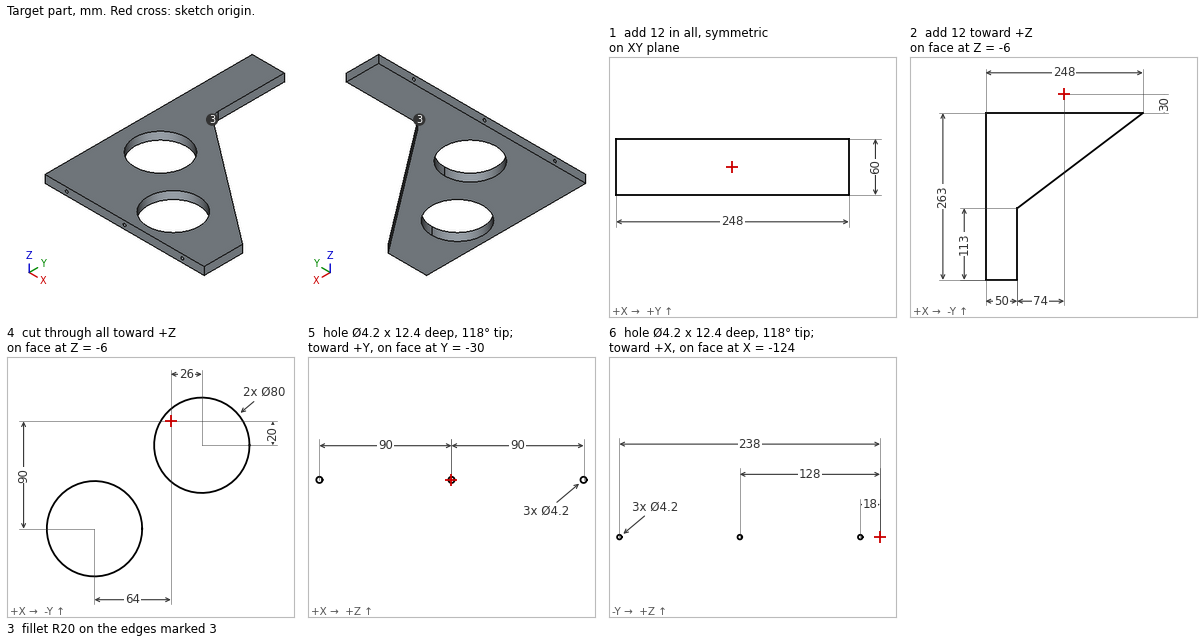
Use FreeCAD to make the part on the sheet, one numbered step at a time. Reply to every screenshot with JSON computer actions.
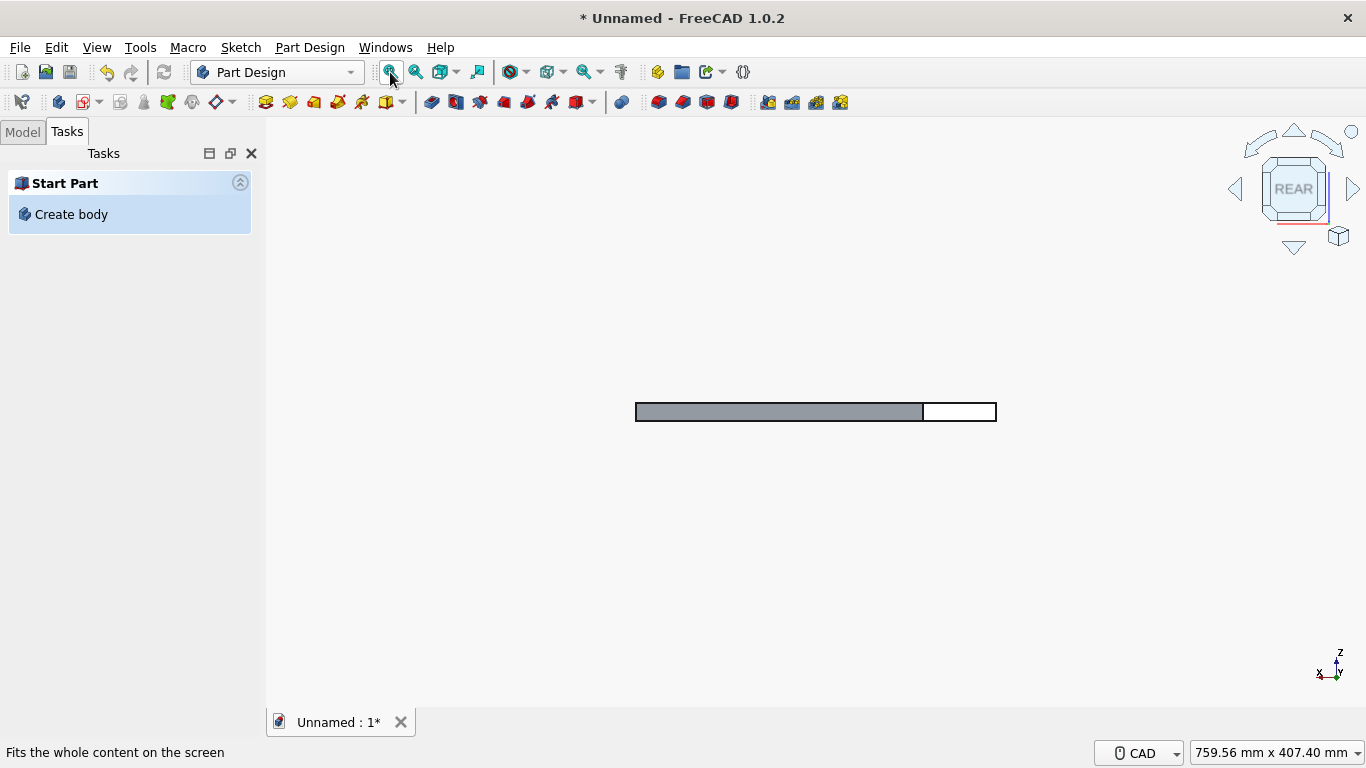
{"action": "scroll", "coordinate": [923, 411], "scroll_direction": "up", "scroll_amount": 5}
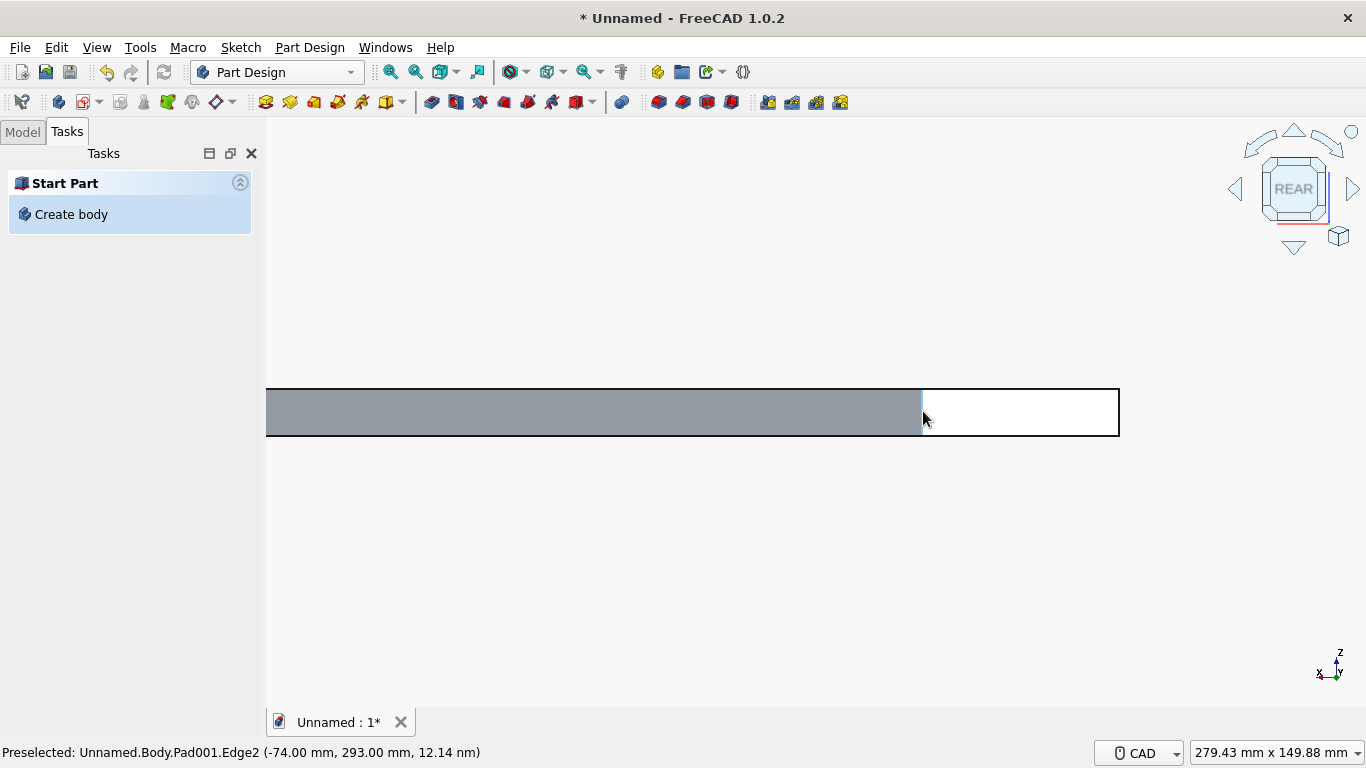
{"action": "left_click", "coordinate": [392, 72]}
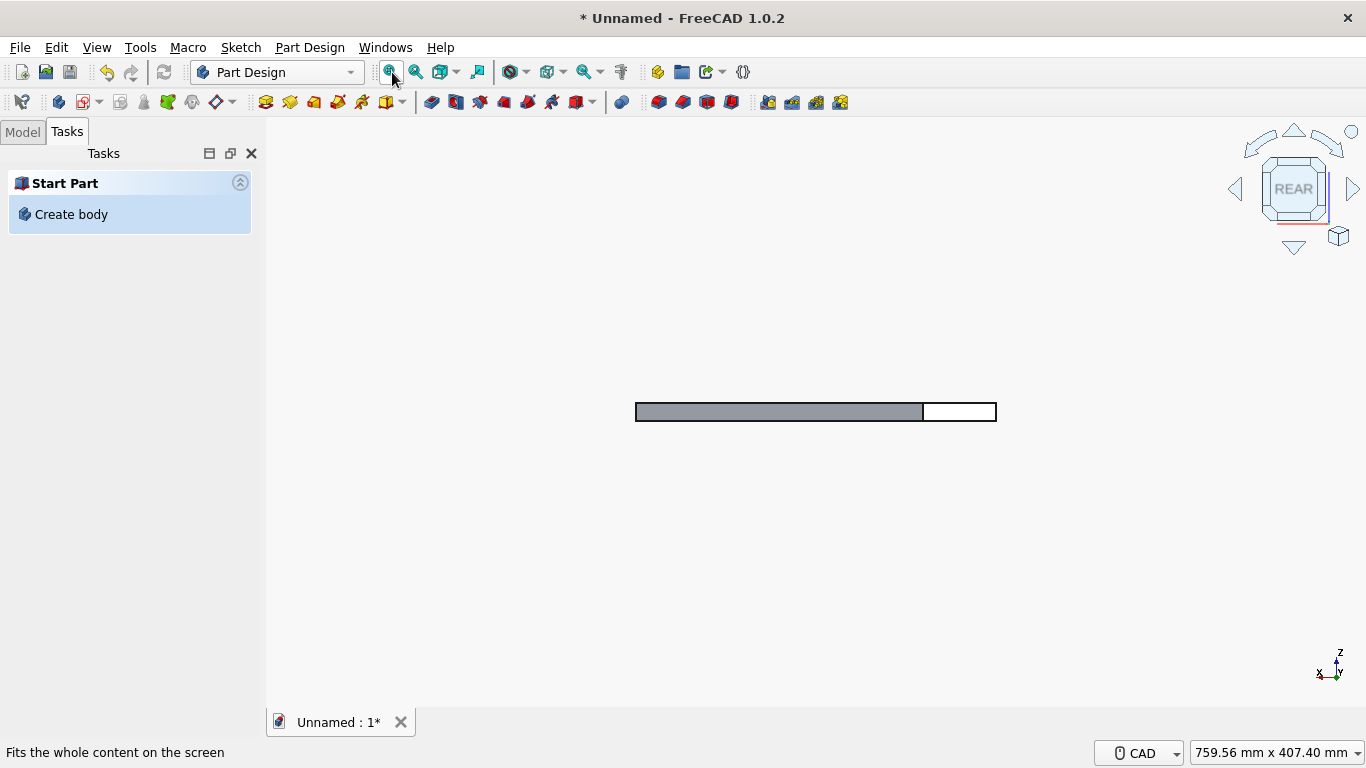
{"action": "key", "text": "6"}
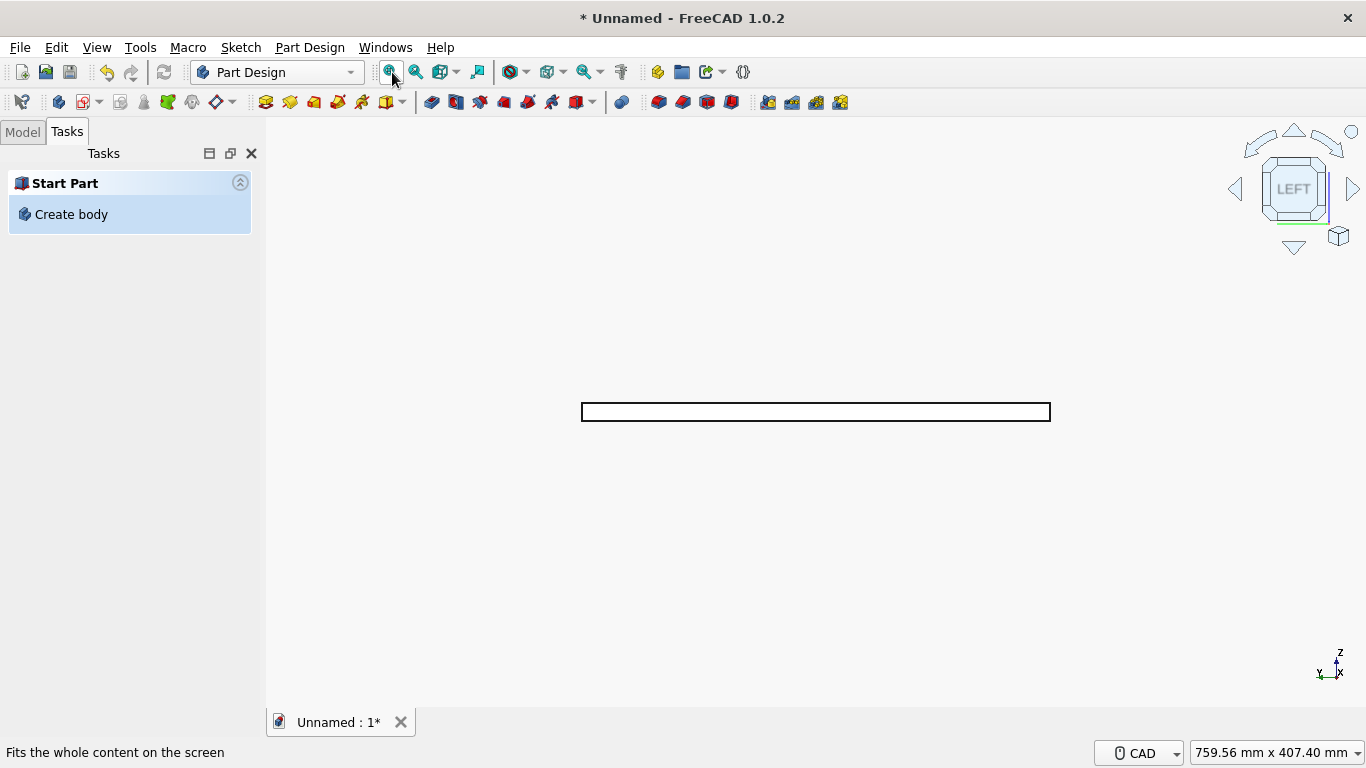
{"action": "key", "text": "v f"}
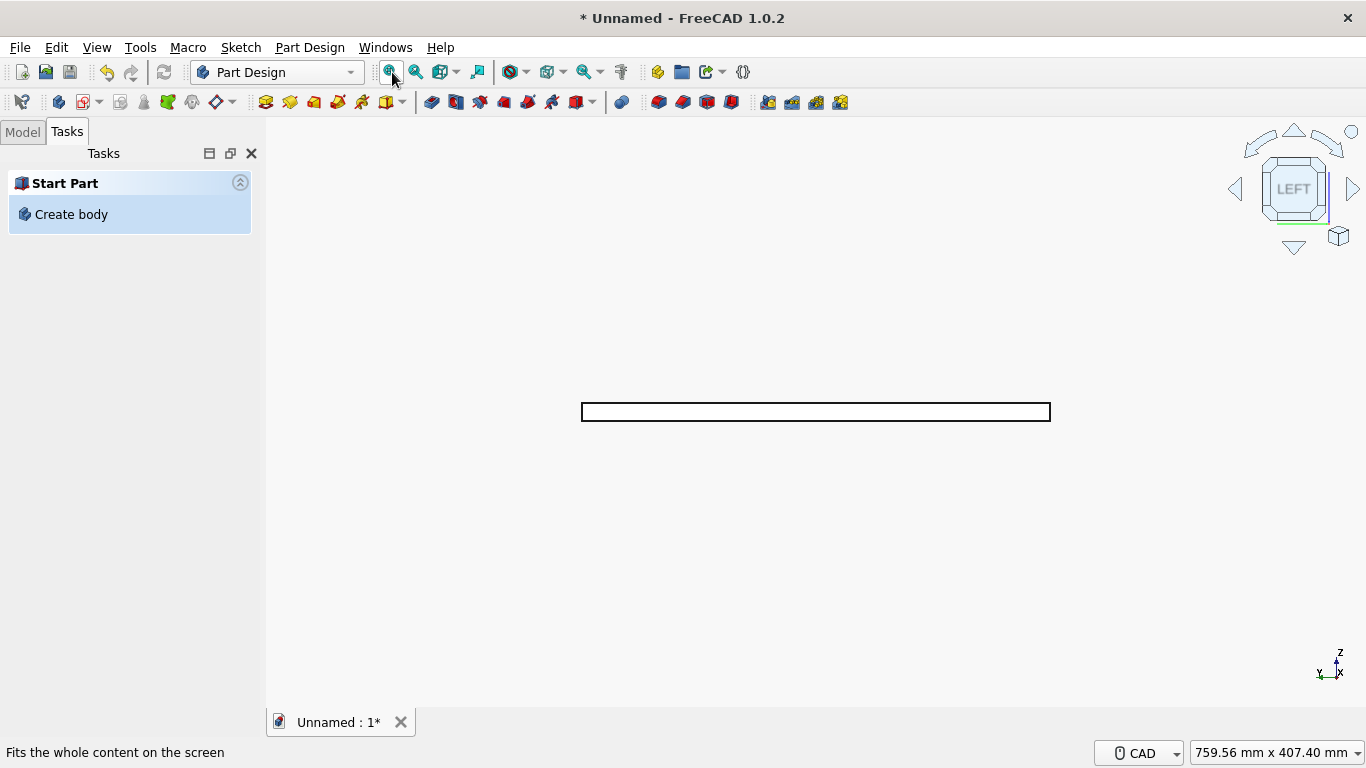
{"action": "scroll", "coordinate": [746, 411], "scroll_direction": "up", "scroll_amount": 5}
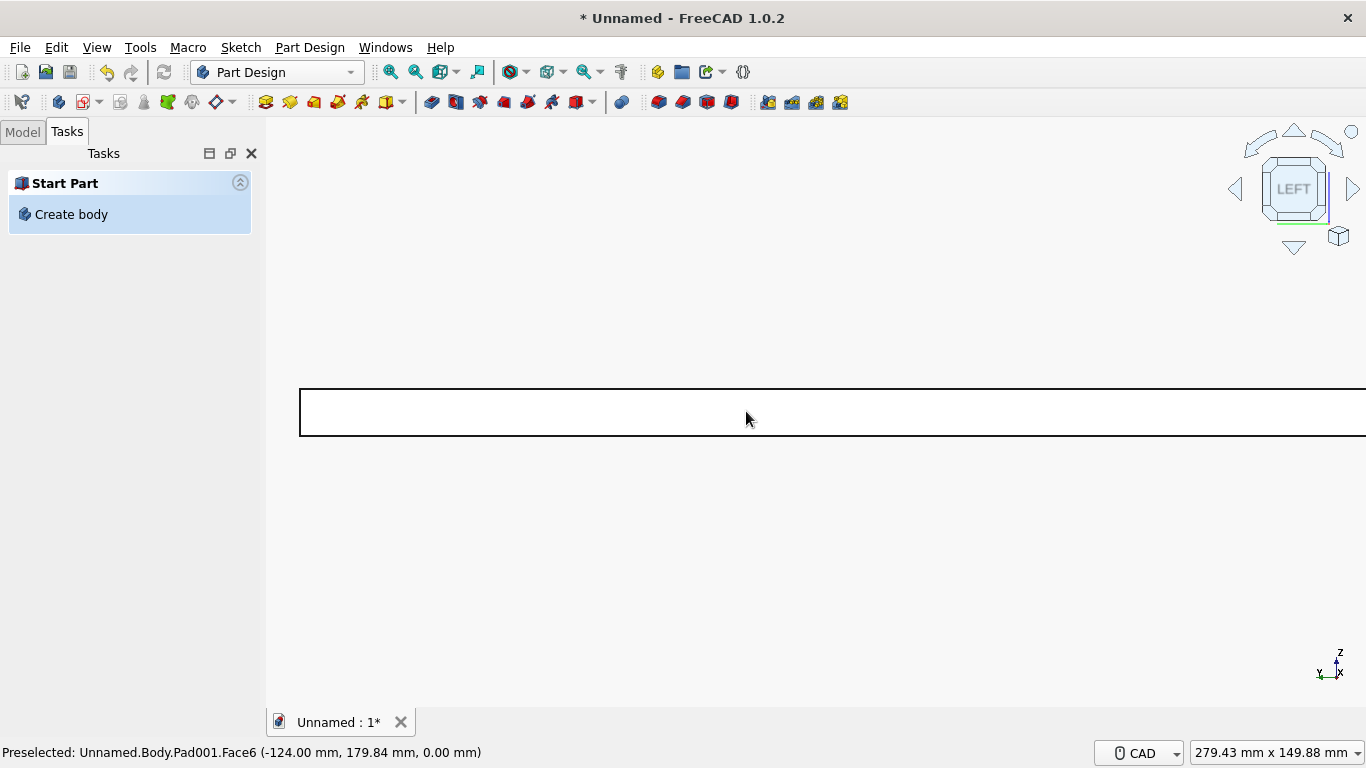
{"action": "key", "text": "v f"}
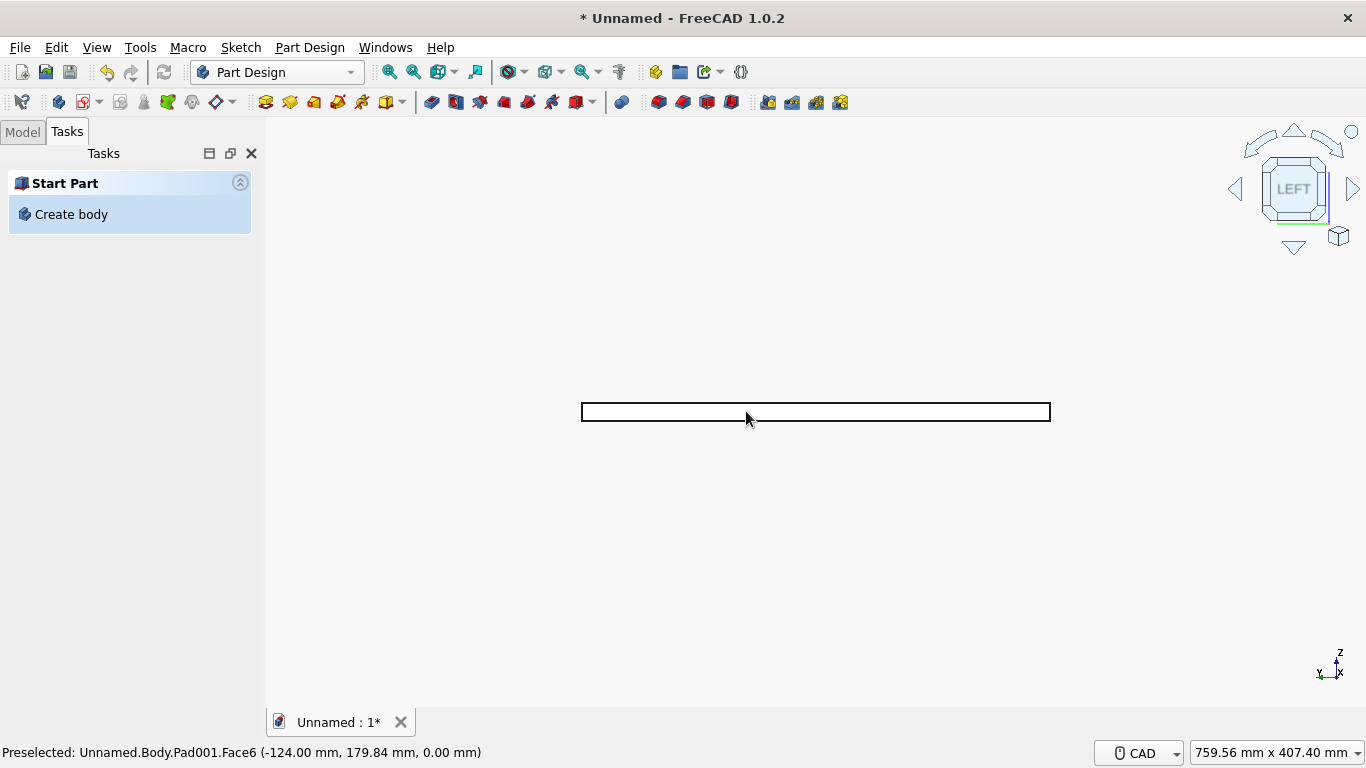
{"action": "key", "text": "v 3"}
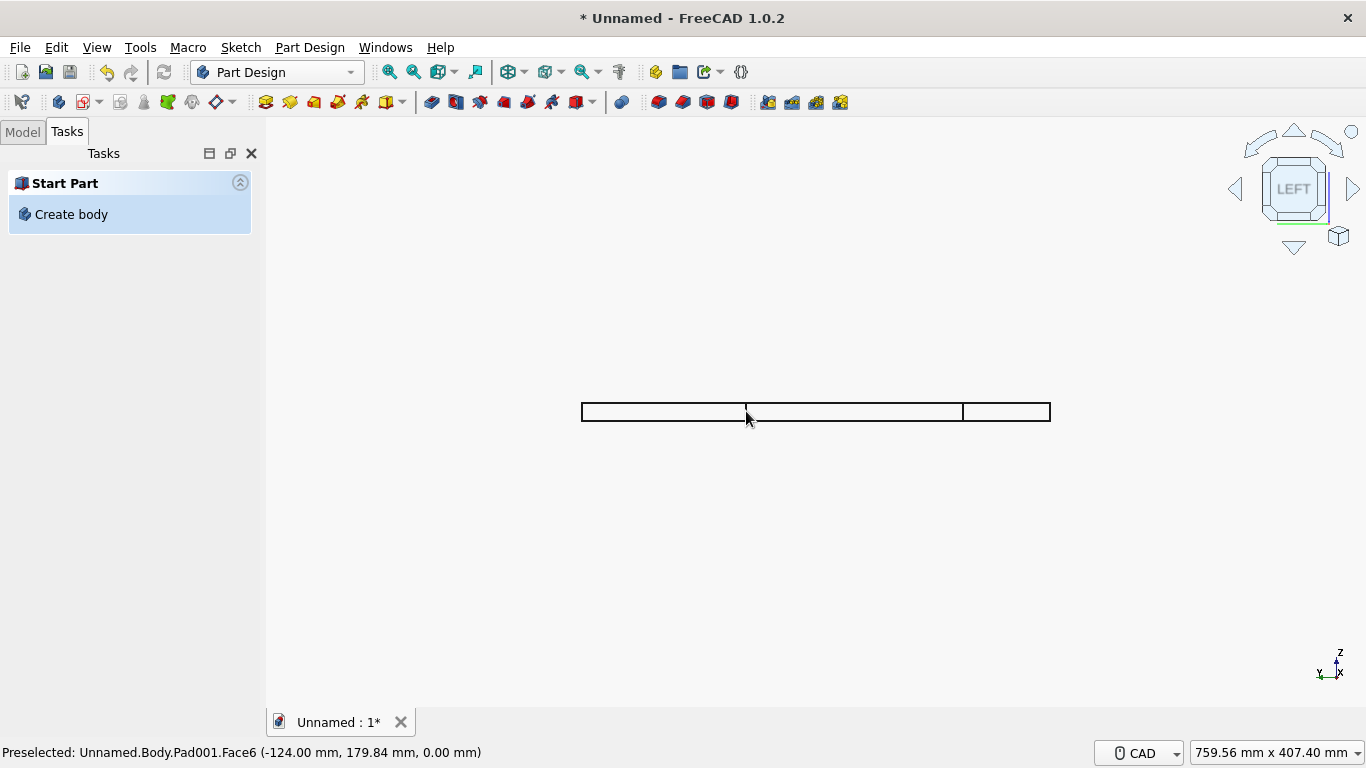
{"action": "key", "text": "0"}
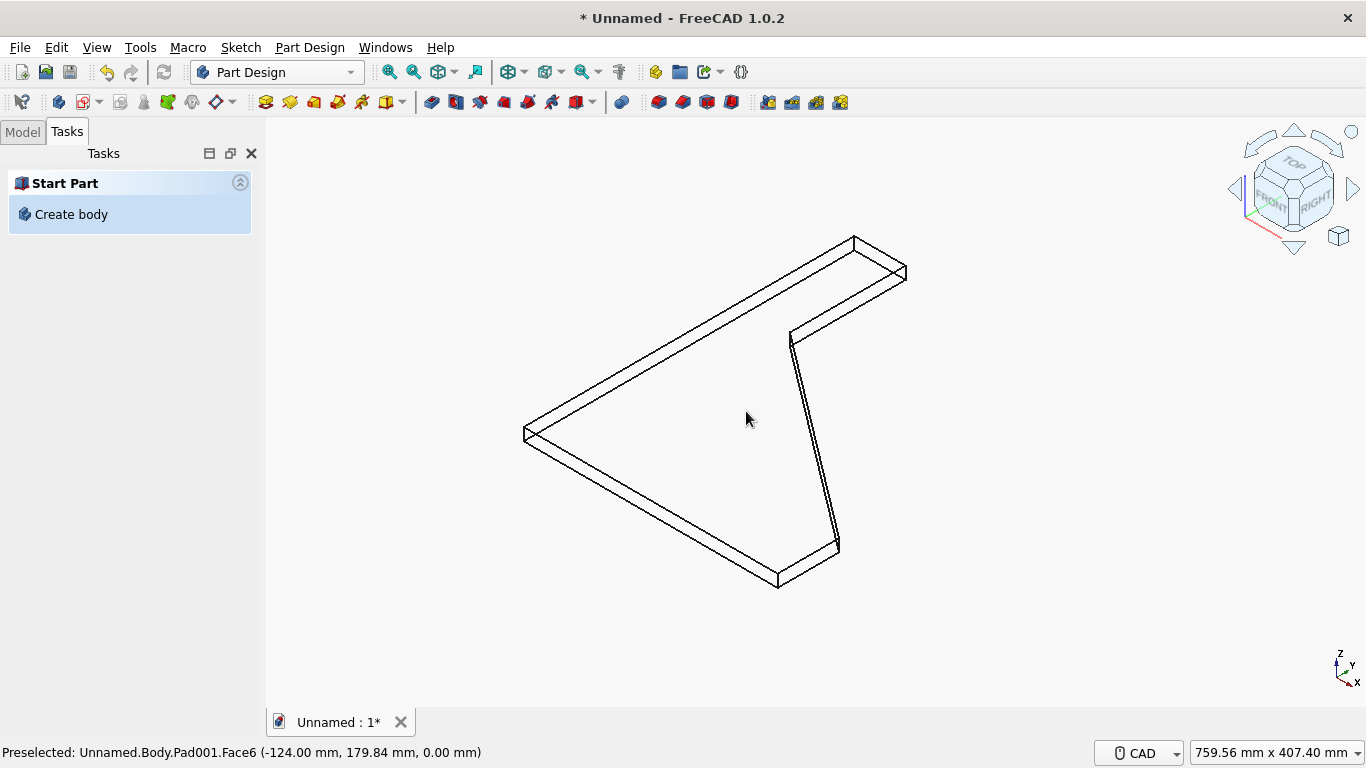
{"action": "scroll", "coordinate": [790, 339], "scroll_direction": "up", "scroll_amount": 6}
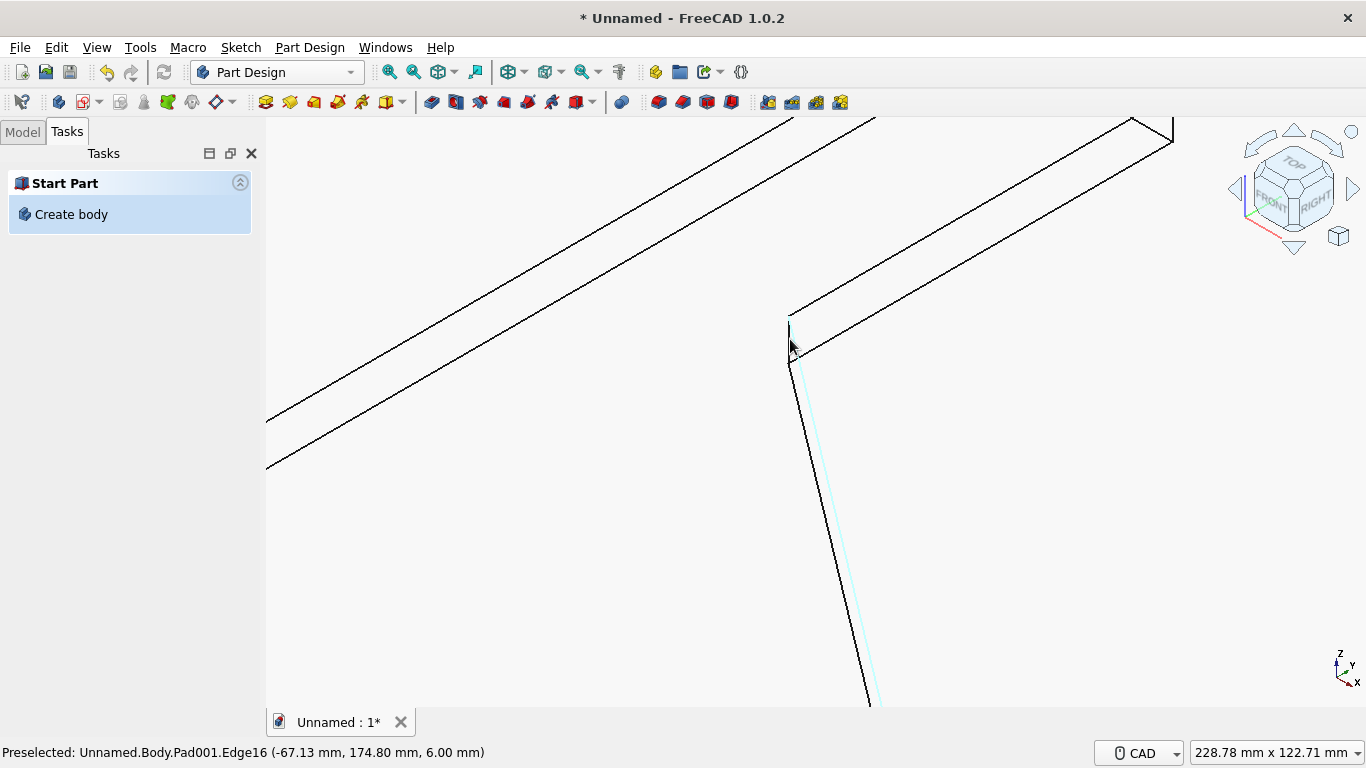
{"action": "left_click", "coordinate": [789, 348]}